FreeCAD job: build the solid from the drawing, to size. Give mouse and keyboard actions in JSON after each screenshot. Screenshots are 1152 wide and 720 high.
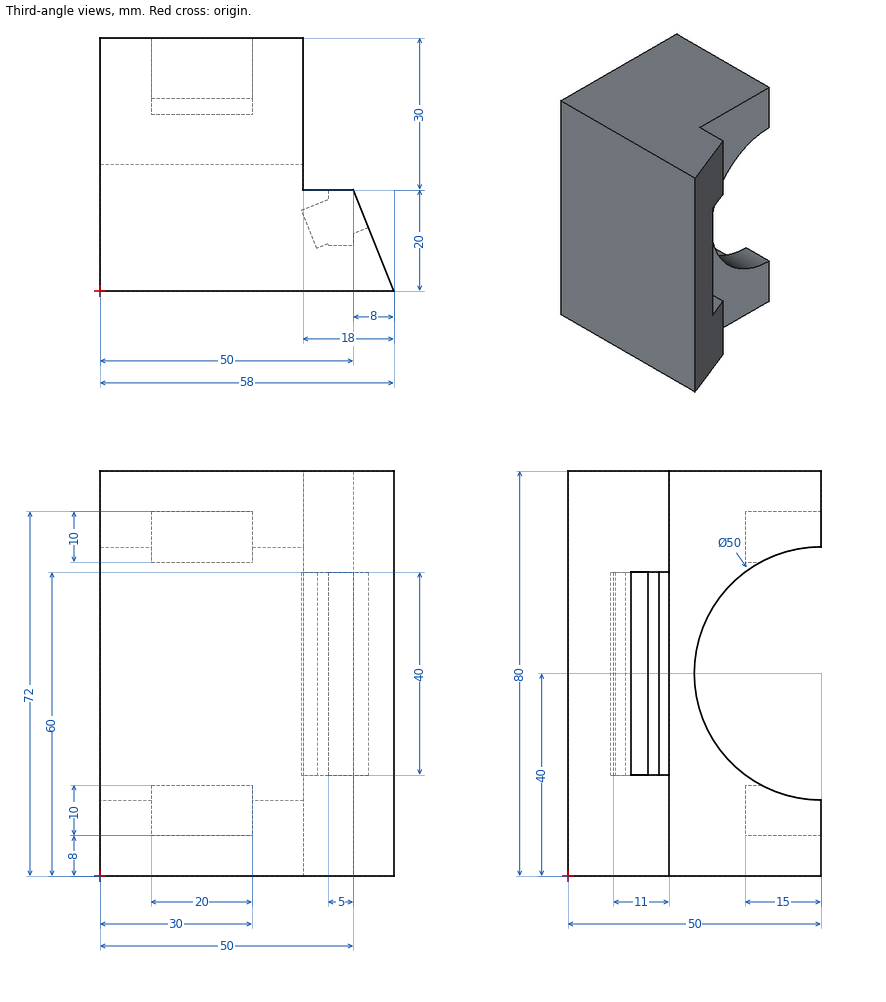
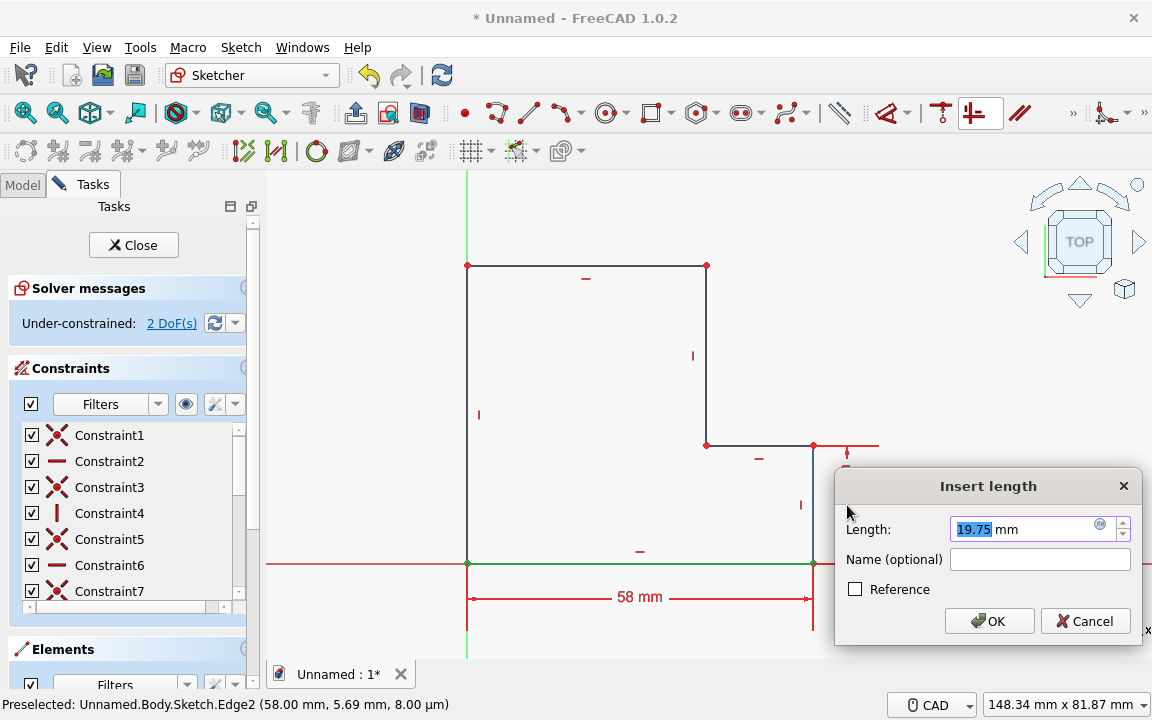
{"action": "type", "text": "20"}
{"action": "key", "text": "Return"}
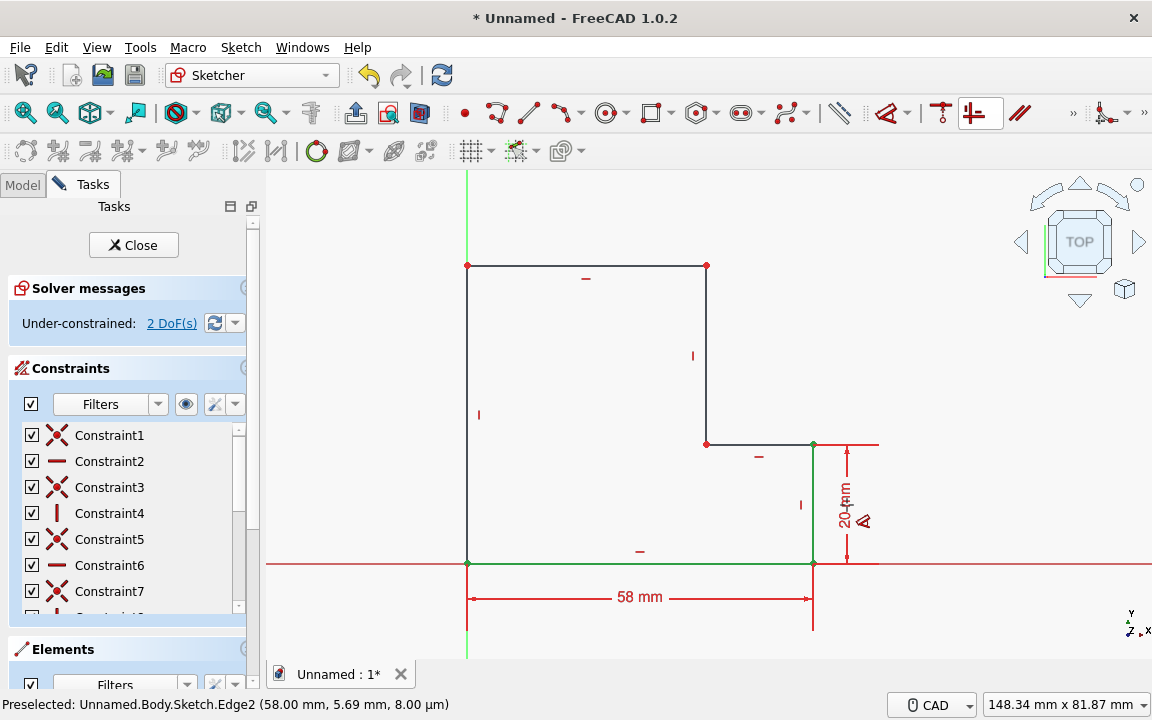
{"action": "left_click", "coordinate": [781, 445]}
{"action": "left_click", "coordinate": [760, 479]}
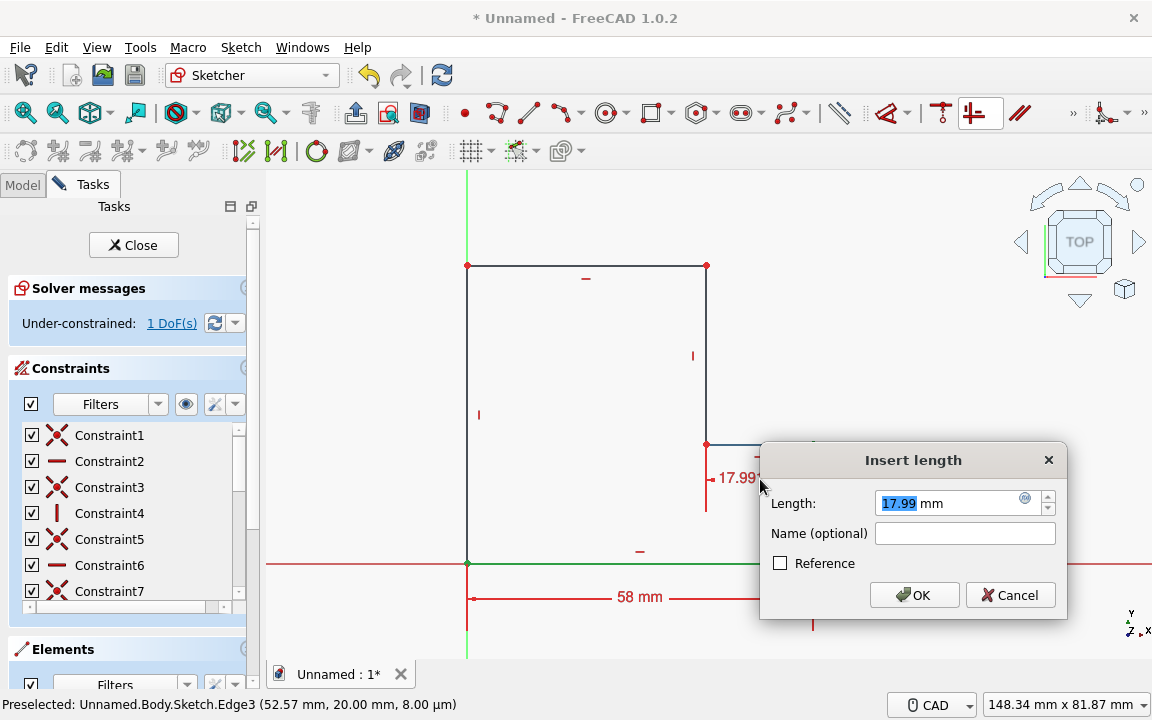
{"action": "type", "text": "18"}
{"action": "key", "text": "Return"}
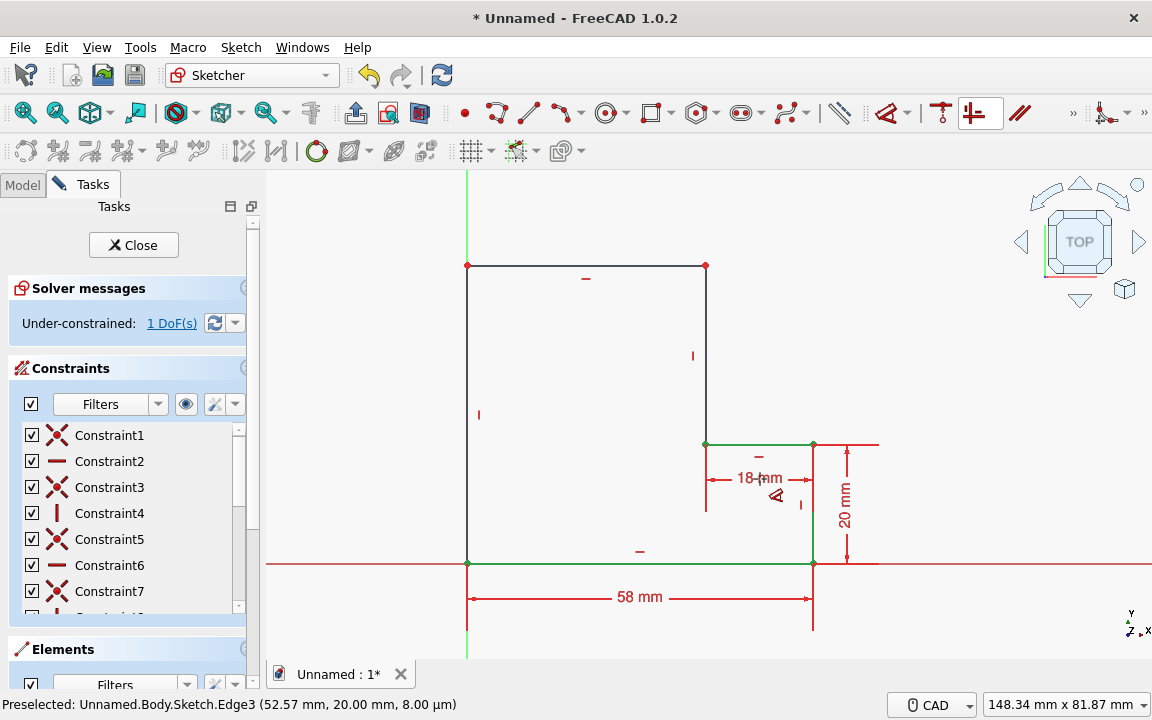
{"action": "left_click", "coordinate": [706, 391]}
{"action": "left_click", "coordinate": [740, 355]}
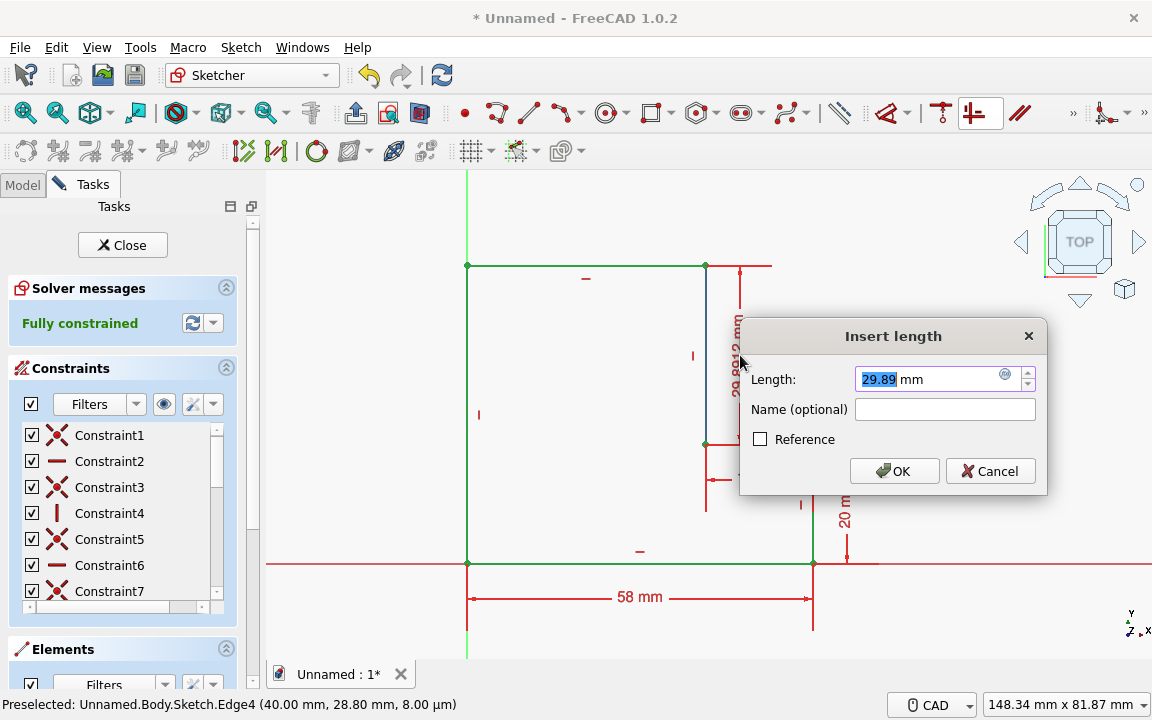
{"action": "type", "text": "30"}
{"action": "key", "text": "Return"}
{"action": "key", "text": "Escape"}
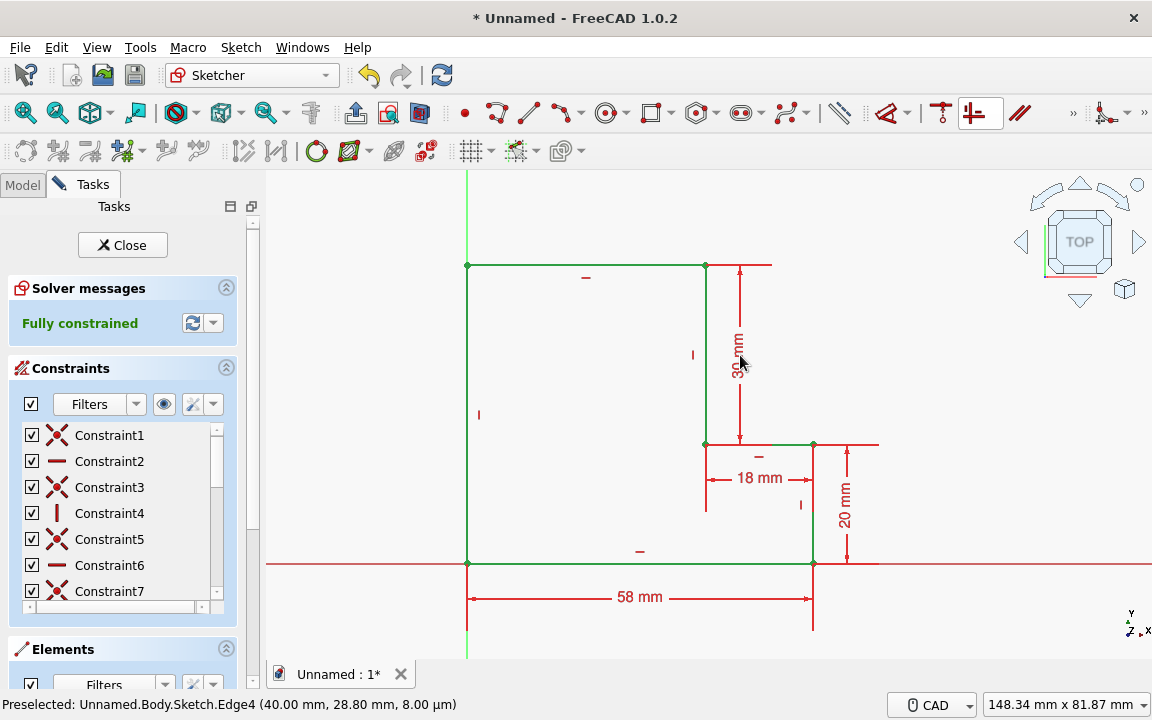
{"action": "left_click", "coordinate": [123, 245]}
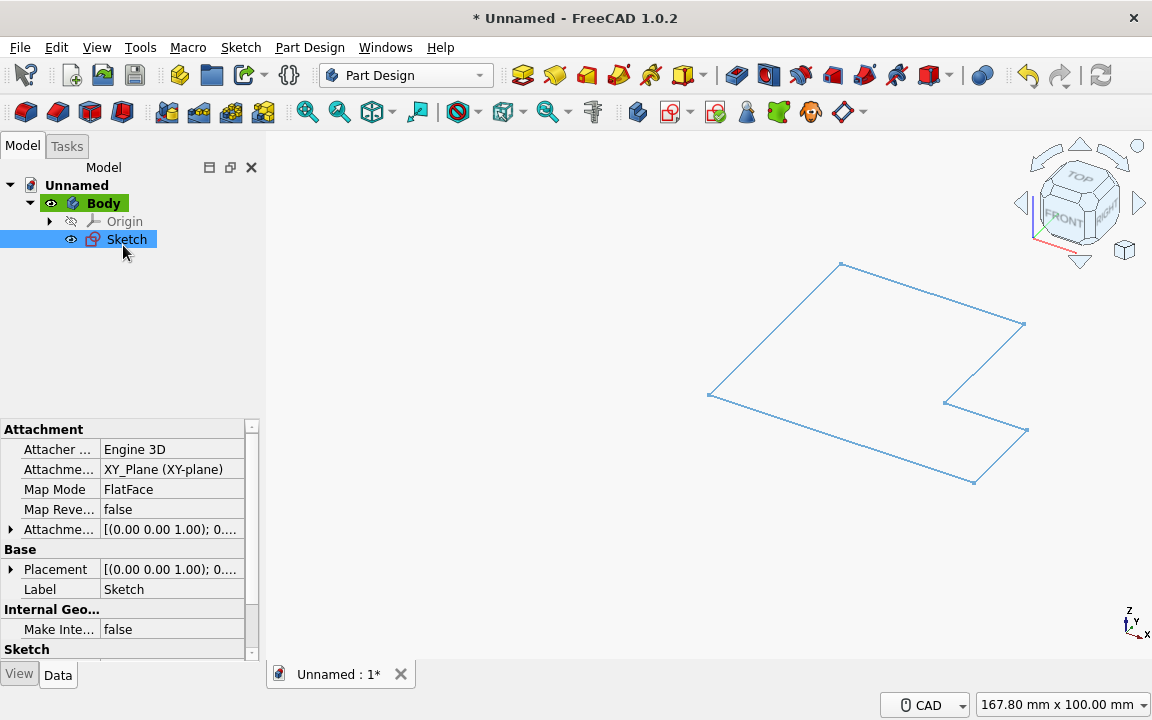
{"action": "left_click", "coordinate": [524, 76]}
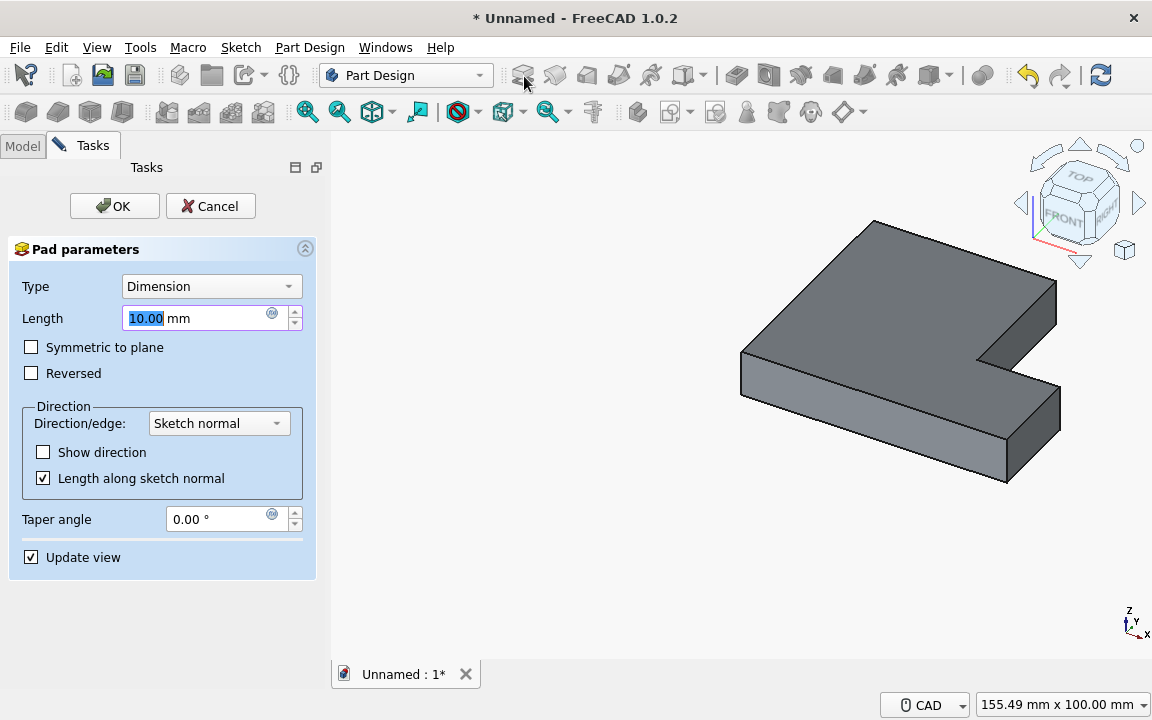
{"action": "type", "text": "80"}
{"action": "key", "text": "Tab"}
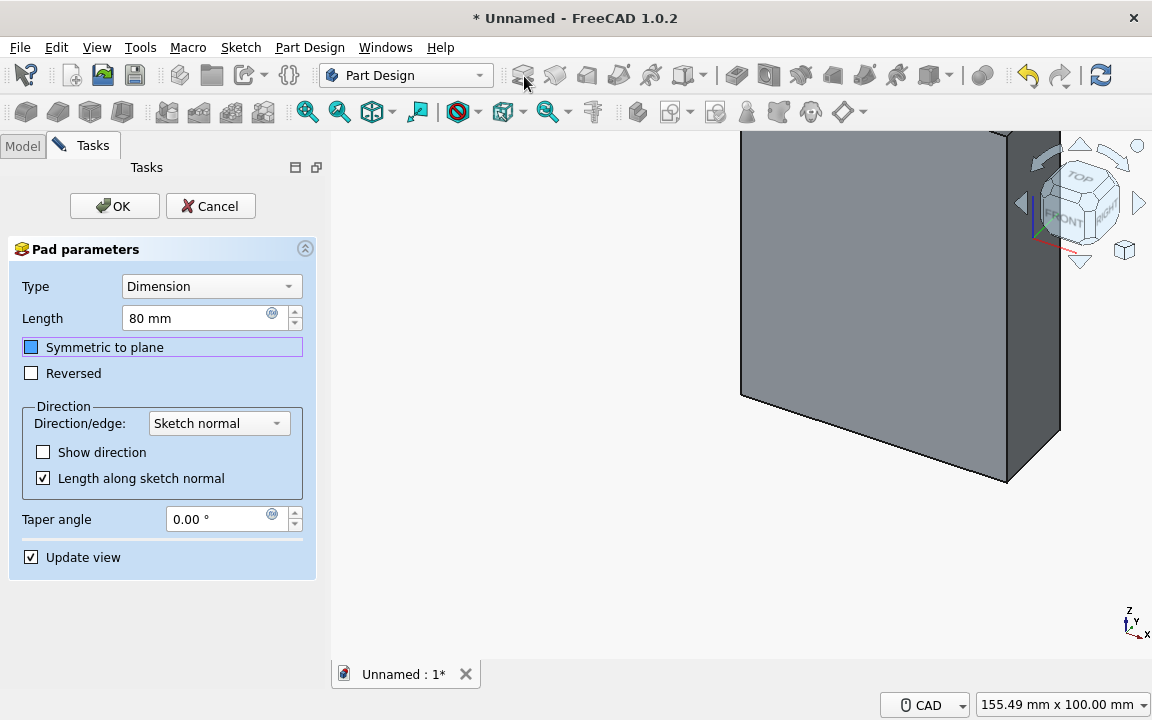
{"action": "left_click", "coordinate": [115, 206]}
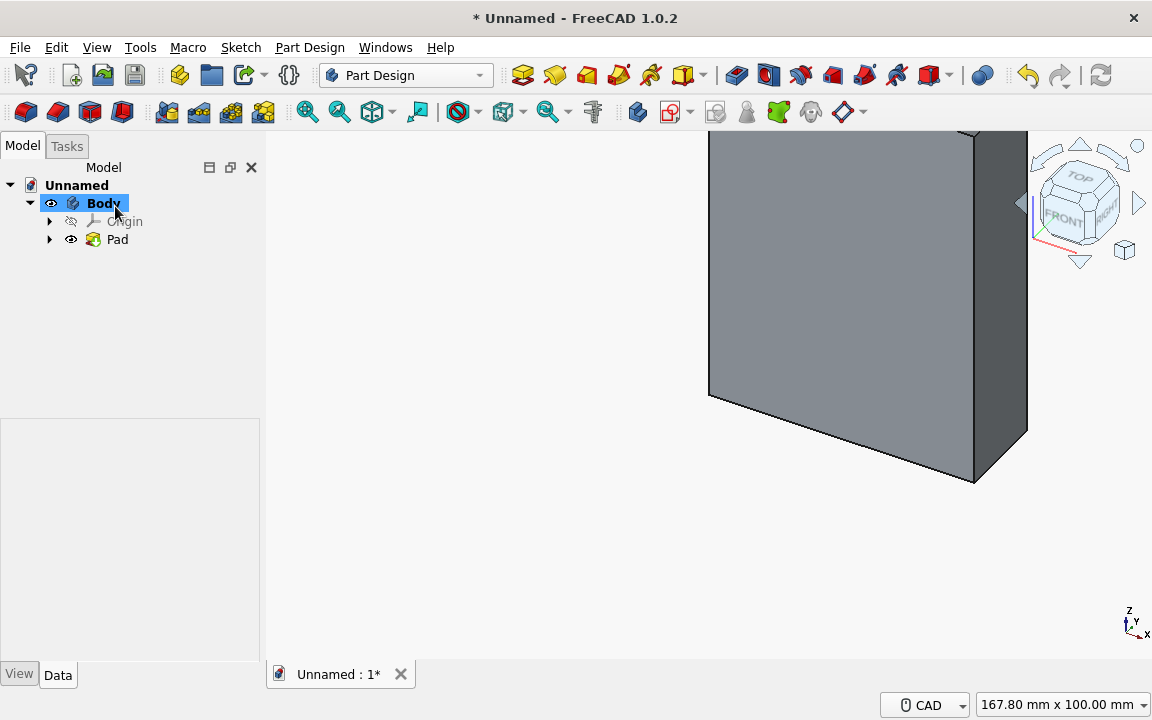
{"action": "left_click", "coordinate": [308, 112]}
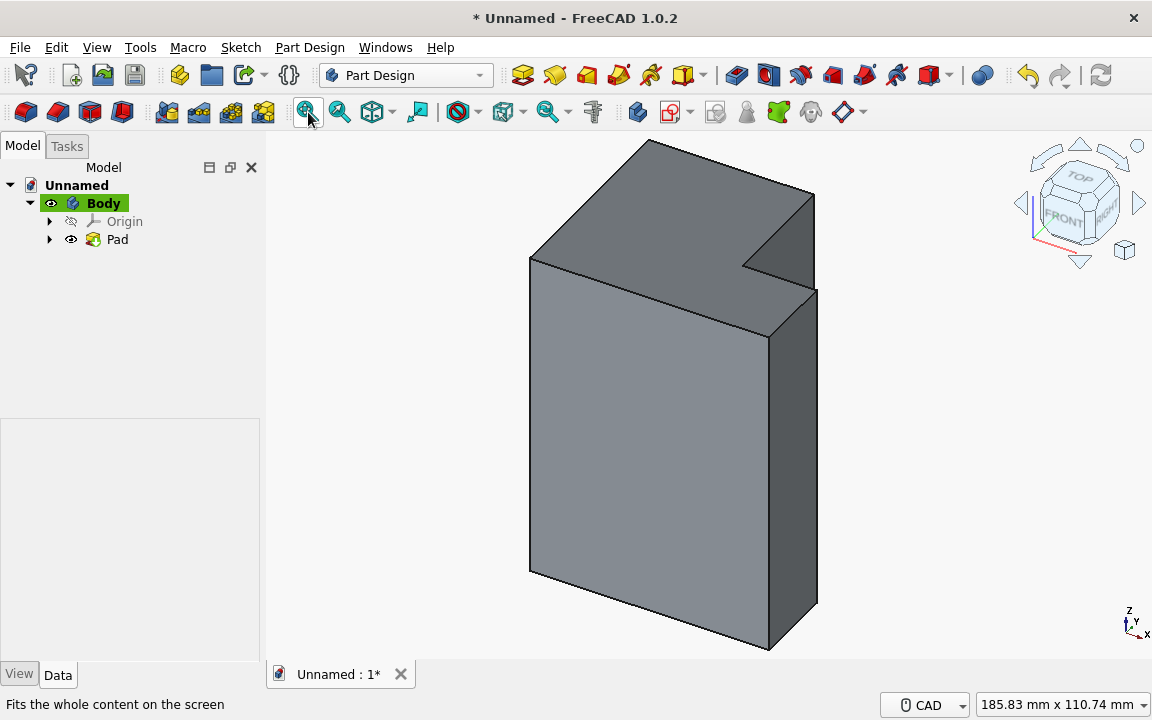
{"action": "key", "text": "4"}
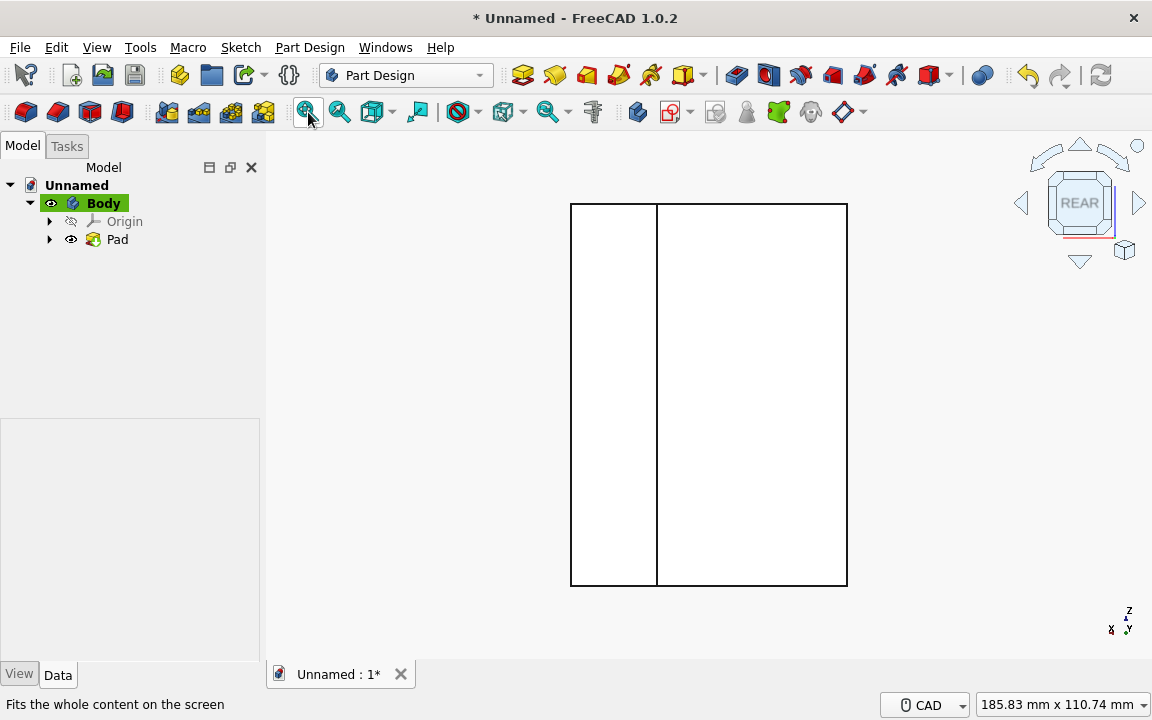
{"action": "left_click", "coordinate": [752, 340]}